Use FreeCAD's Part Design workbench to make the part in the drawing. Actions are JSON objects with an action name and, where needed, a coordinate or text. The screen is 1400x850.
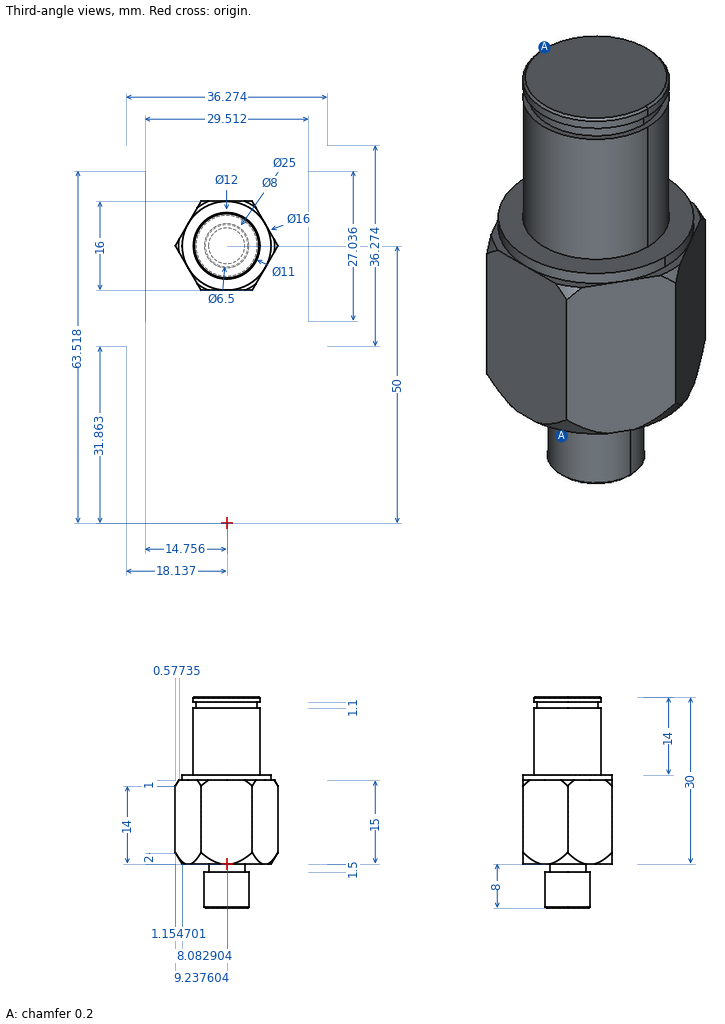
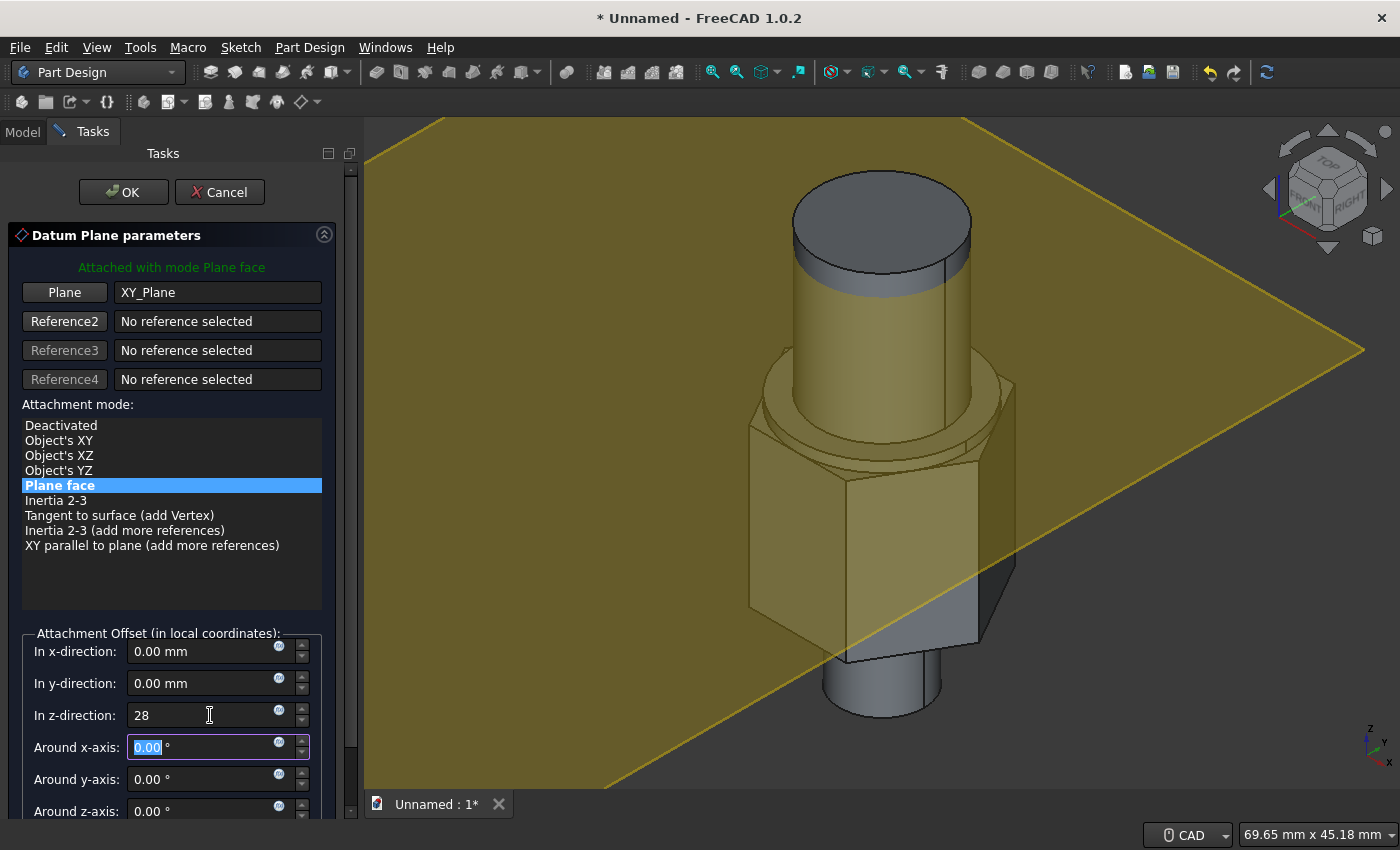
{"action": "left_click", "coordinate": [124, 192]}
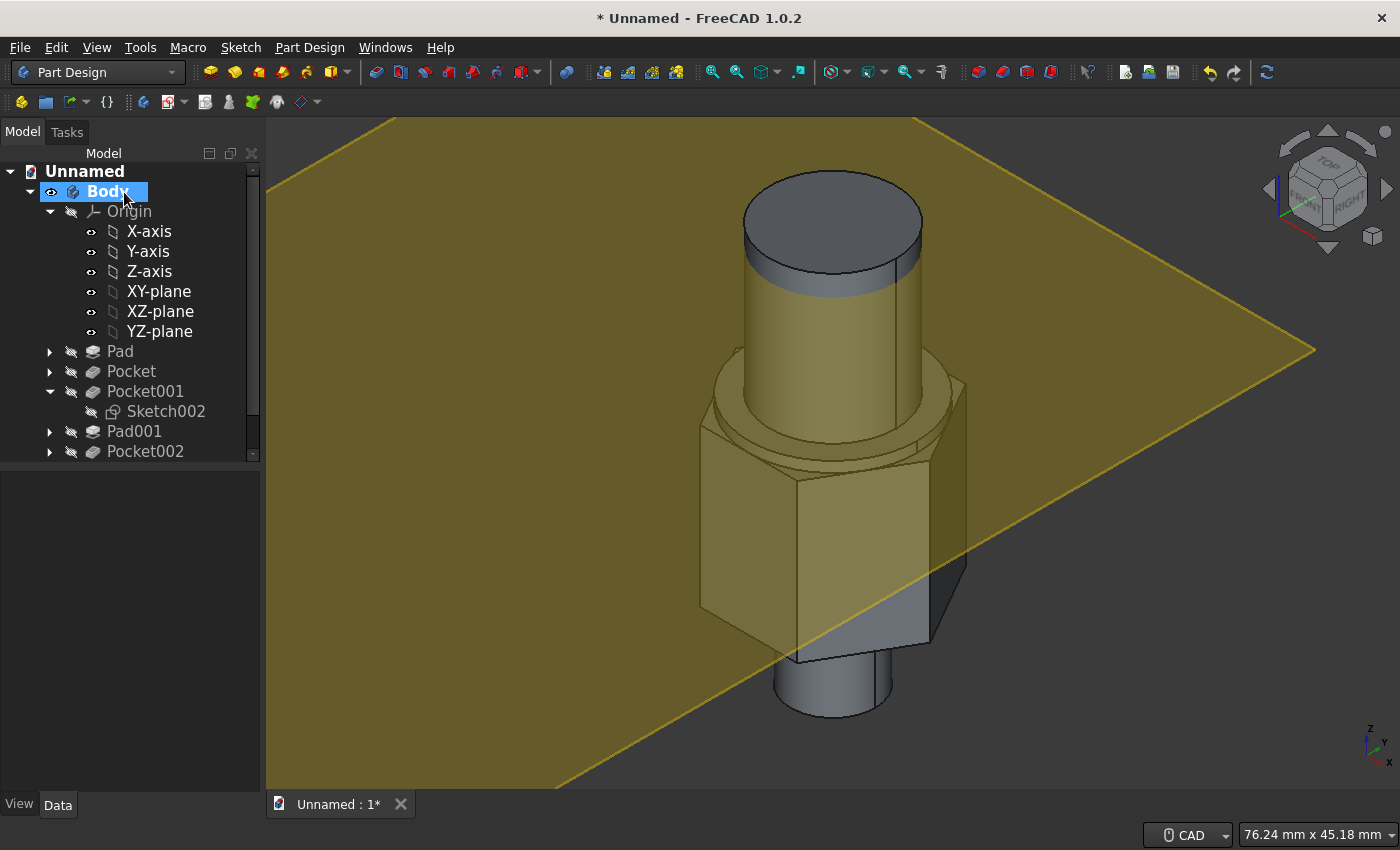
{"action": "scroll", "coordinate": [100, 307], "scroll_direction": "down", "scroll_amount": 3}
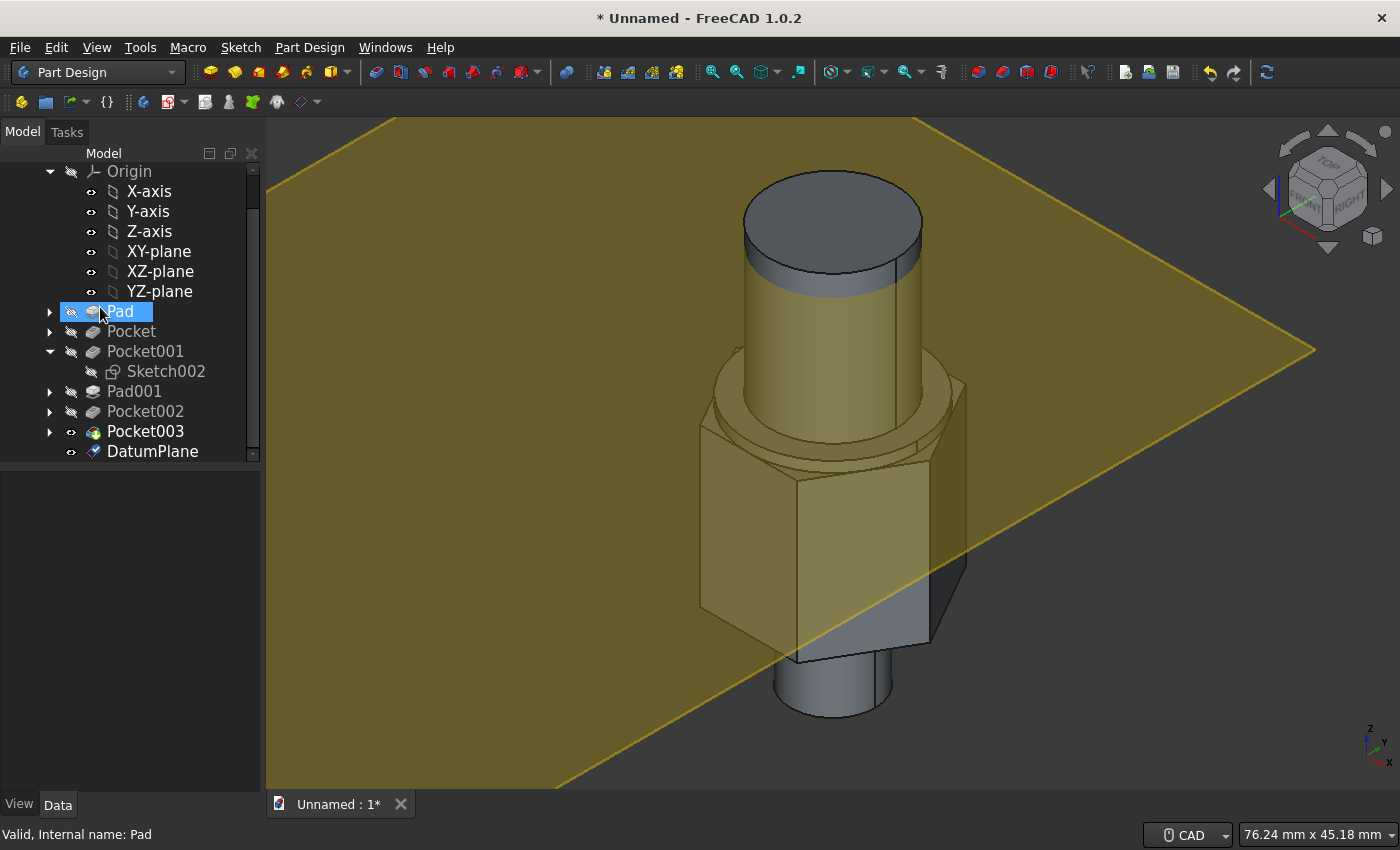
{"action": "left_click", "coordinate": [116, 452]}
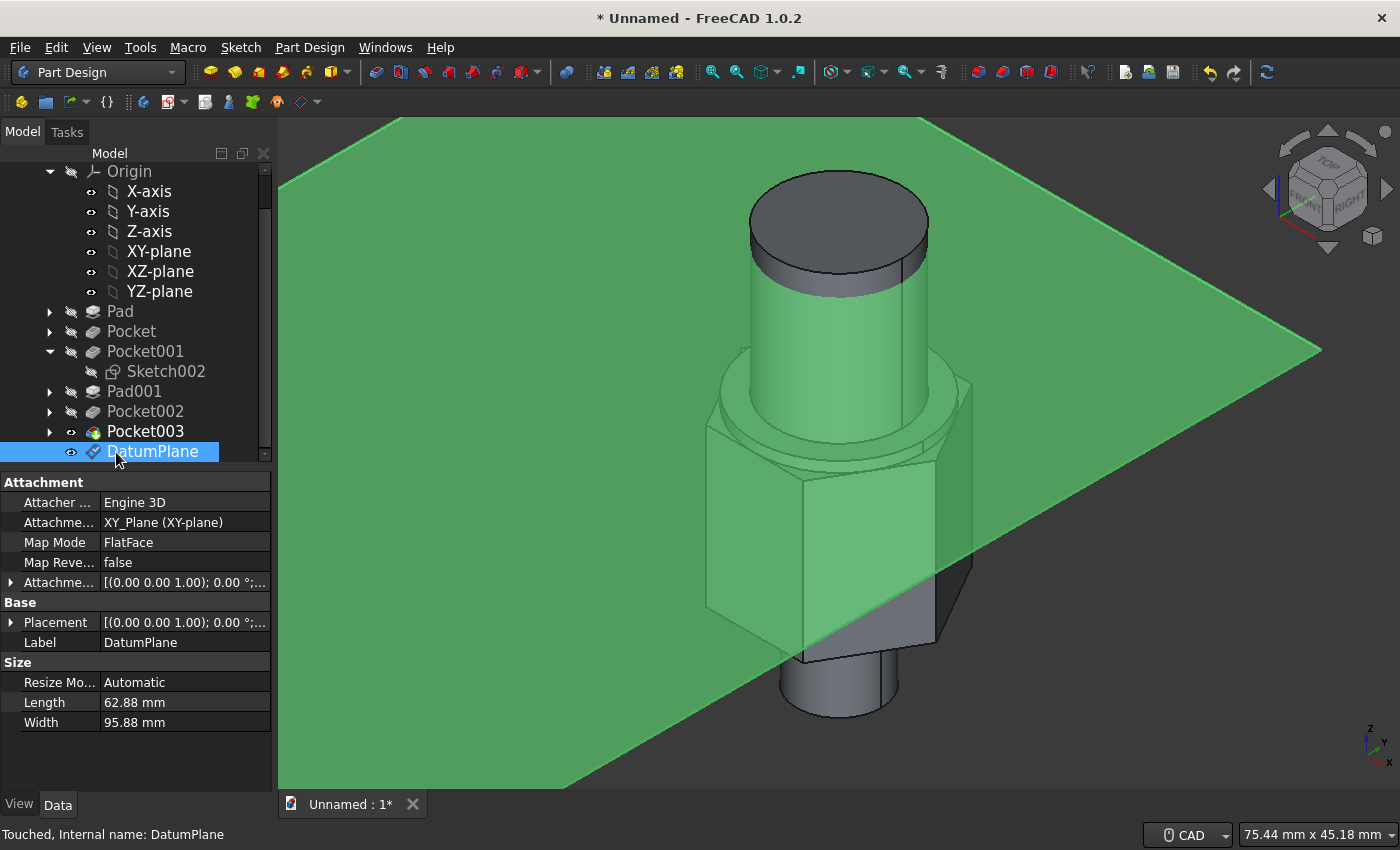
{"action": "left_click", "coordinate": [168, 102]}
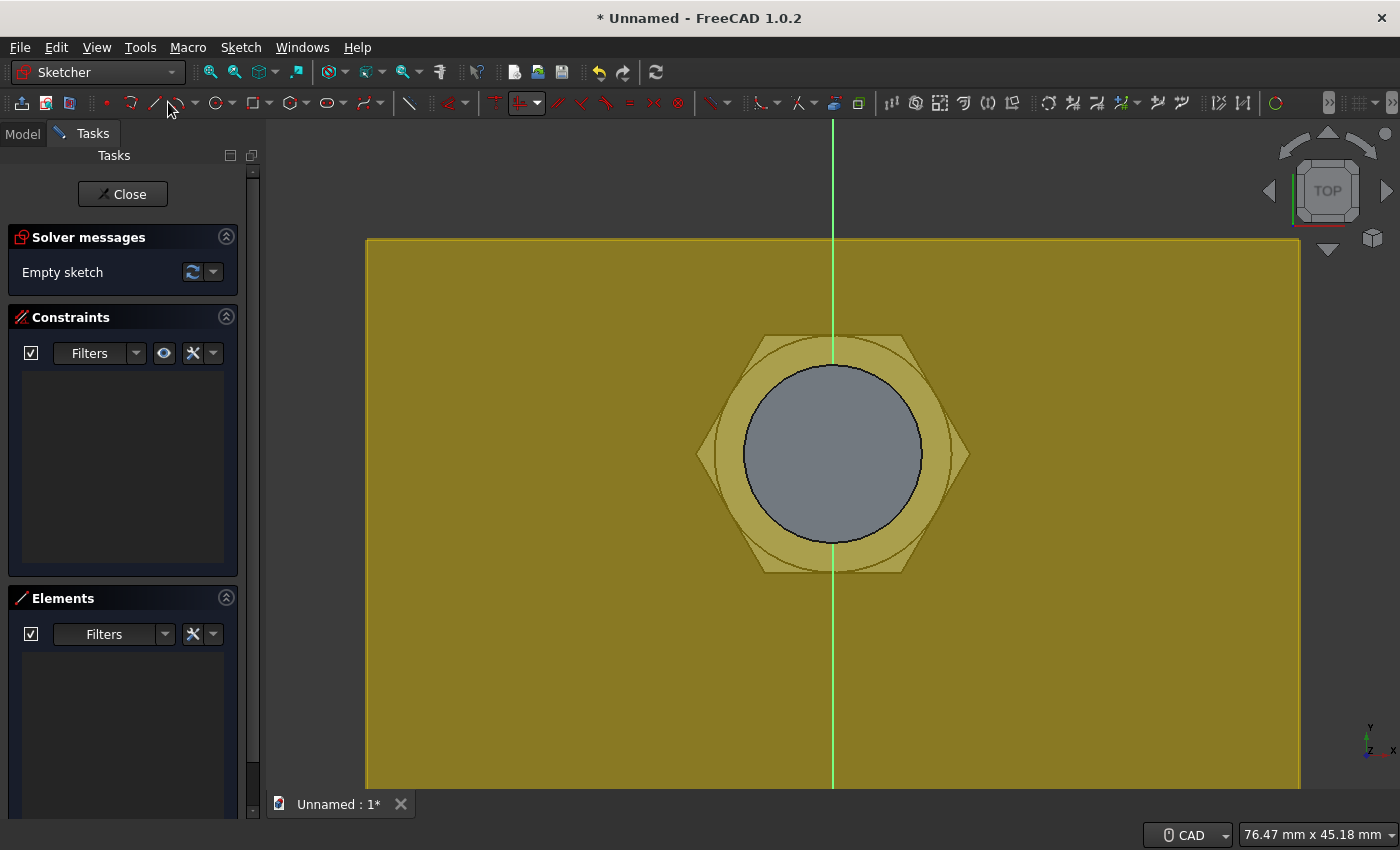
{"action": "left_click", "coordinate": [70, 104]}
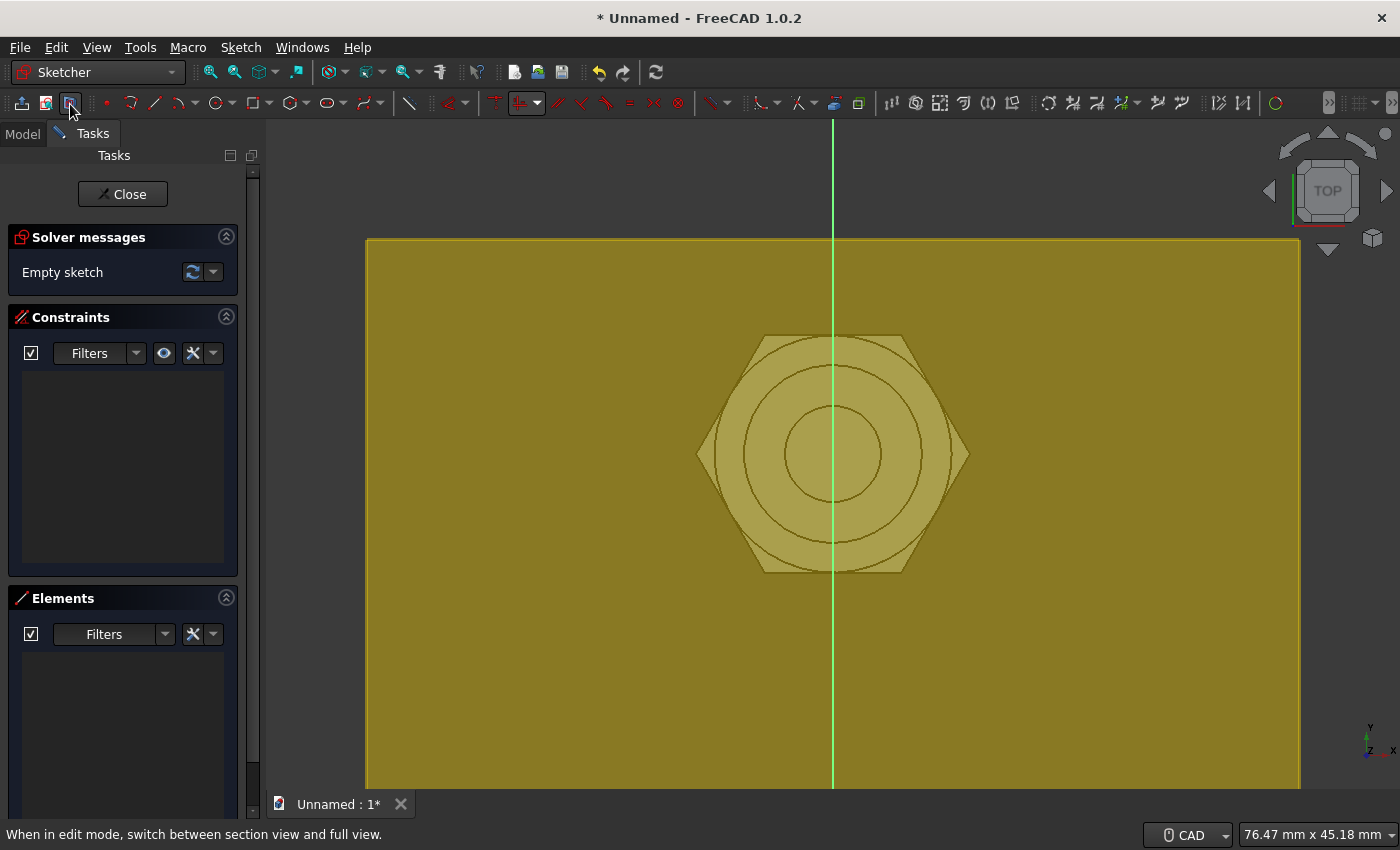
{"action": "scroll", "coordinate": [709, 233], "scroll_direction": "down", "scroll_amount": 4}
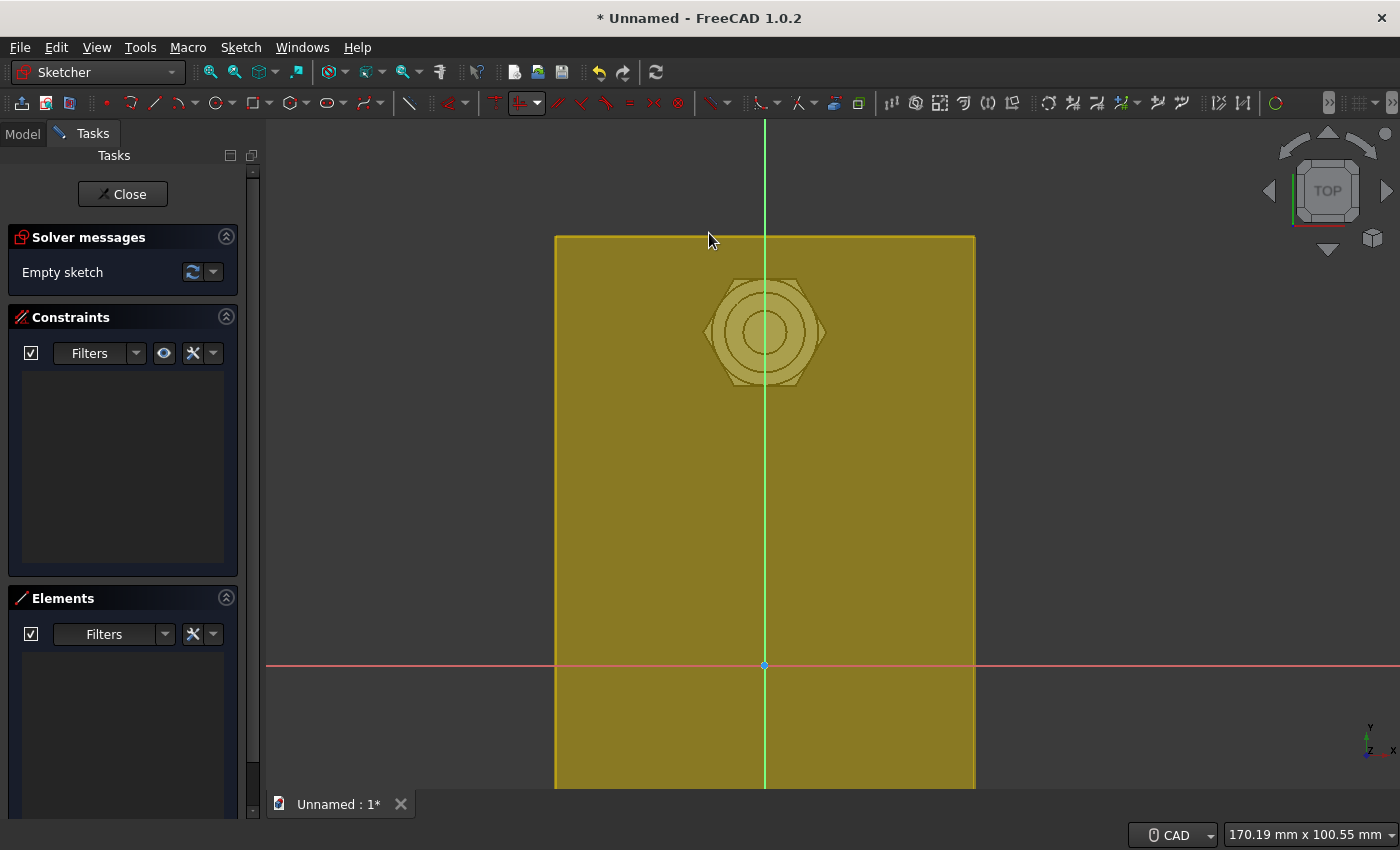
{"action": "left_click", "coordinate": [254, 104]}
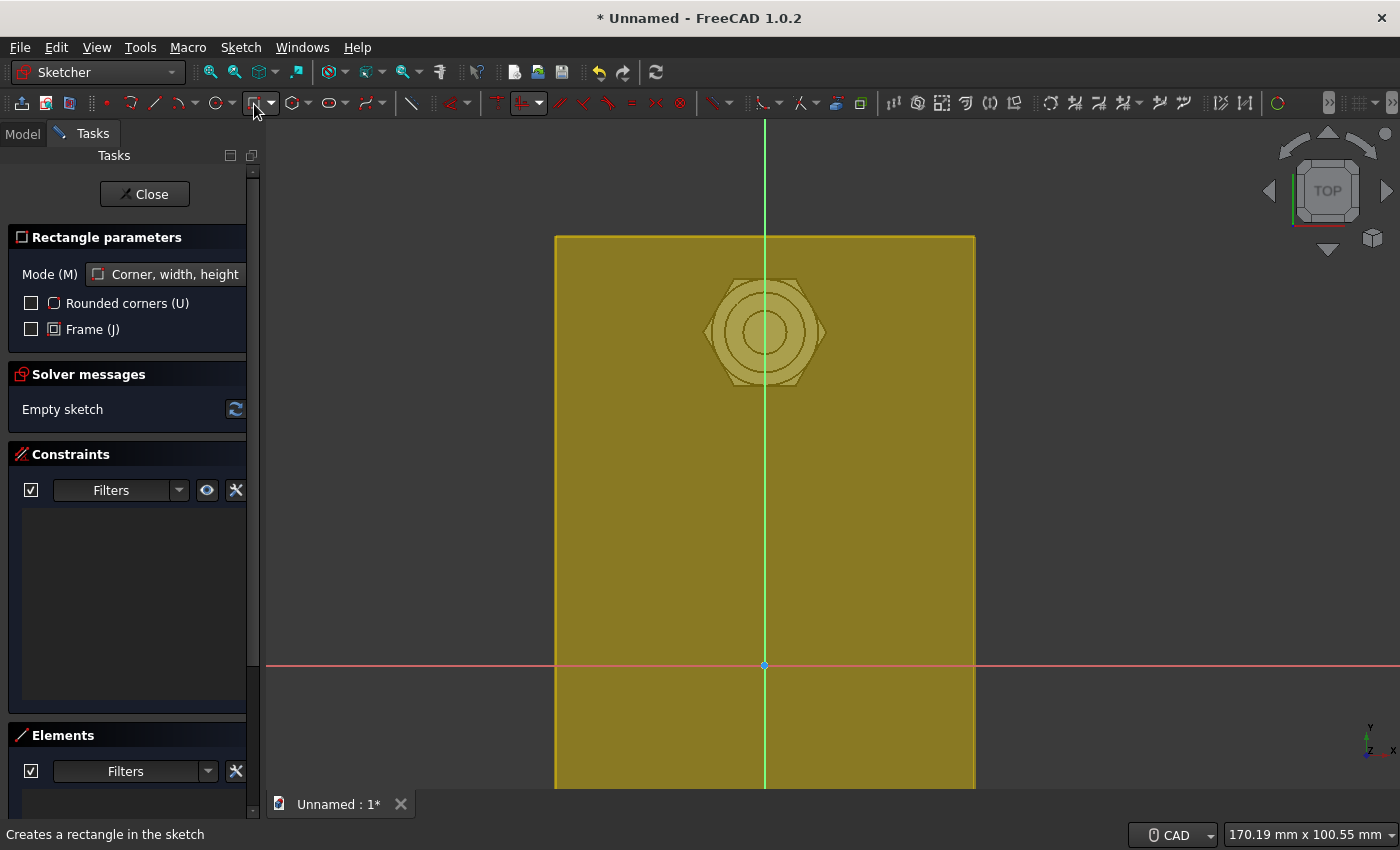
{"action": "left_click", "coordinate": [667, 242]}
{"action": "mouse_move", "coordinate": [863, 422]}